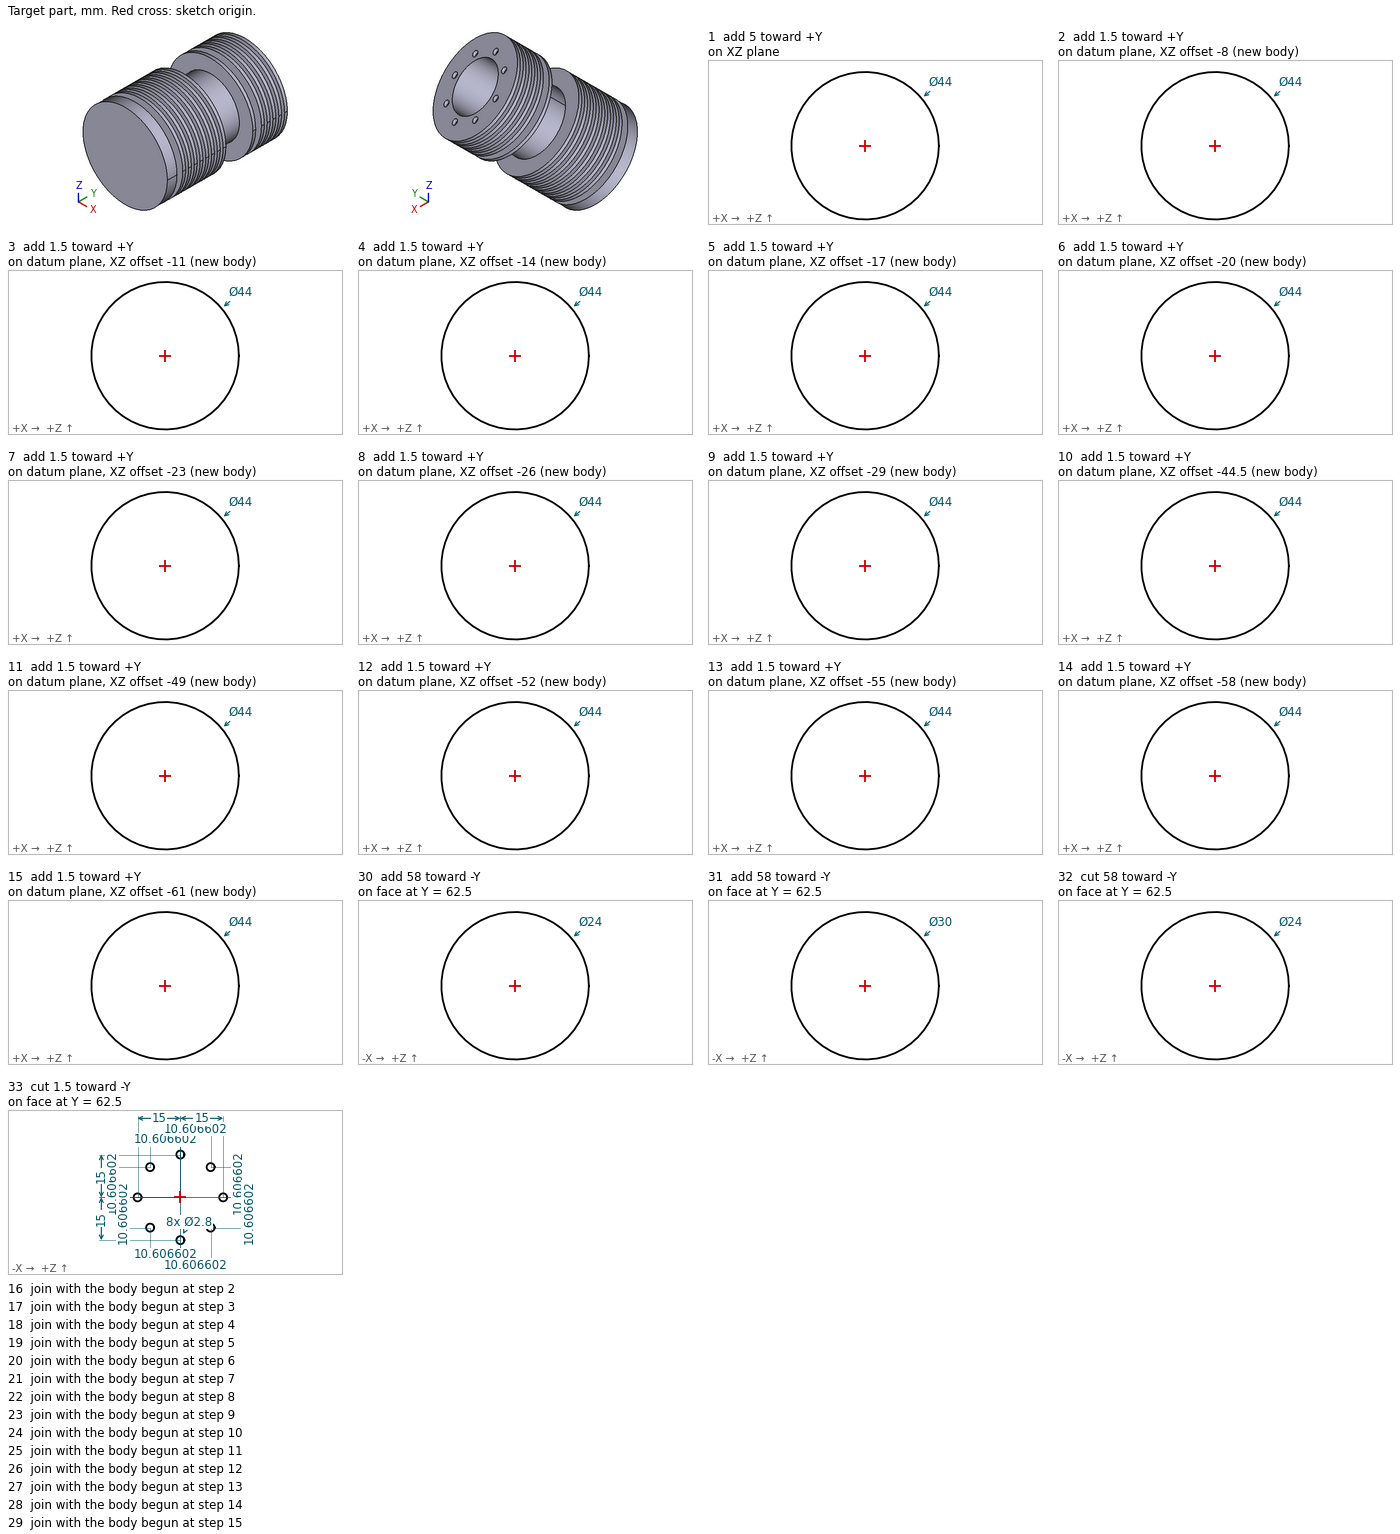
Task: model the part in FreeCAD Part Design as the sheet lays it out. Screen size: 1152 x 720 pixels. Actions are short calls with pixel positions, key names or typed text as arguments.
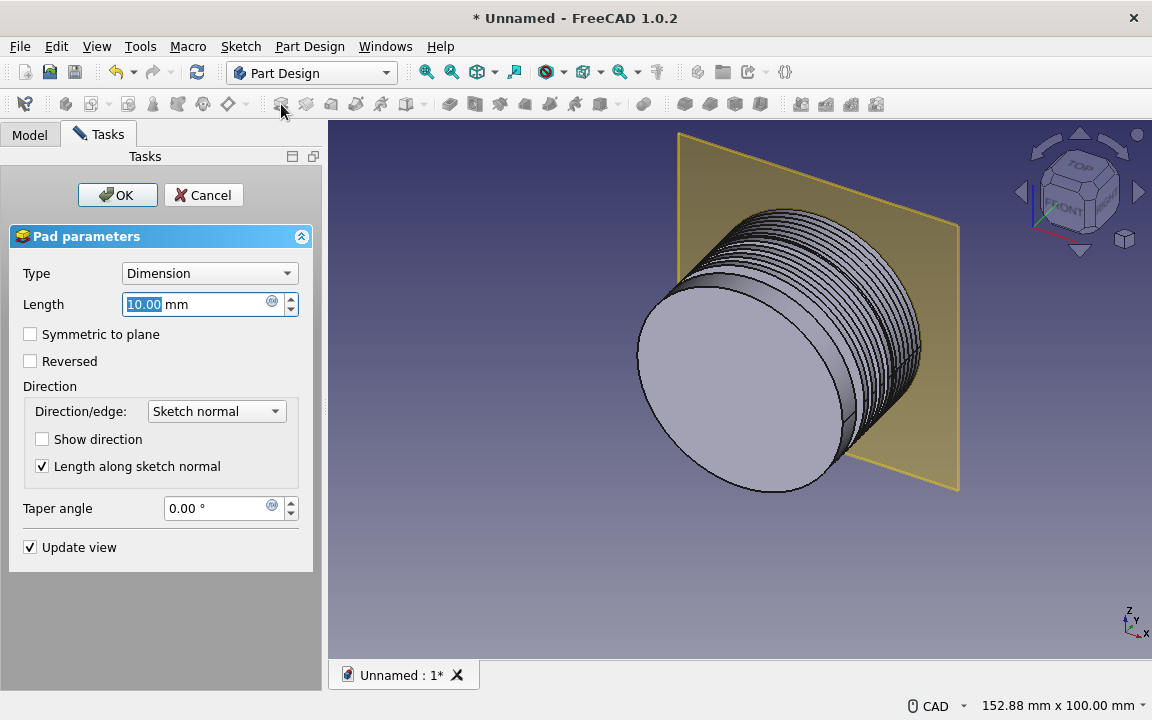
text(1.5)
key(Tab)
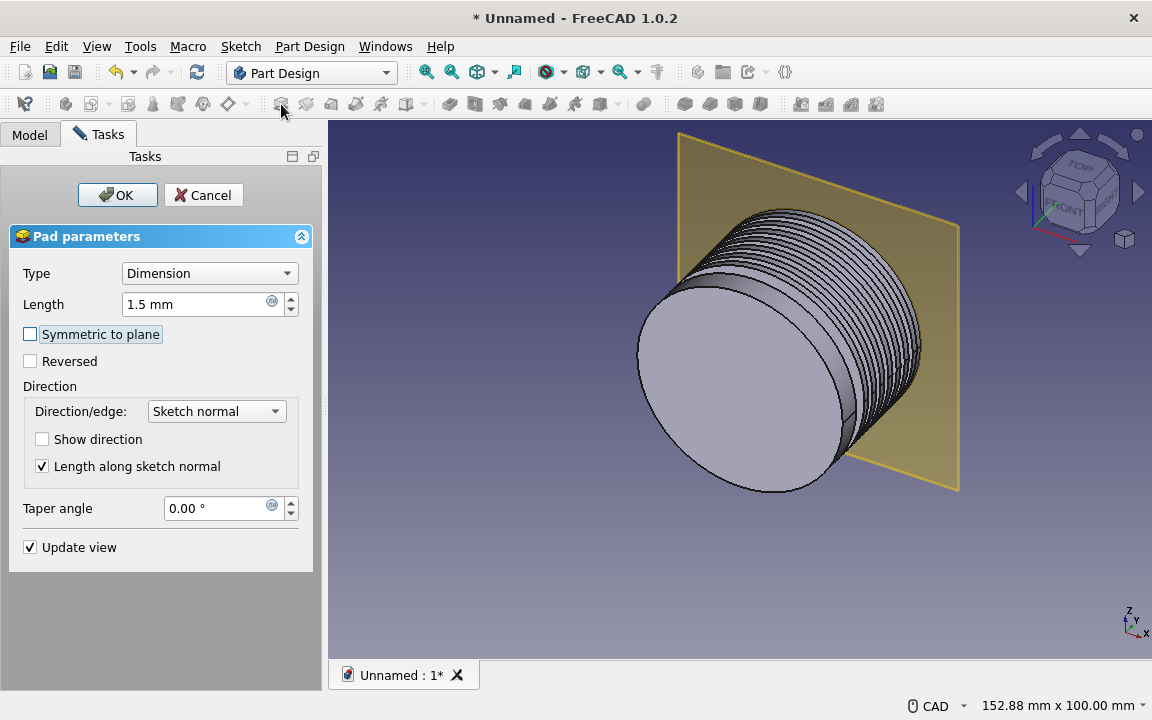
click(31, 361)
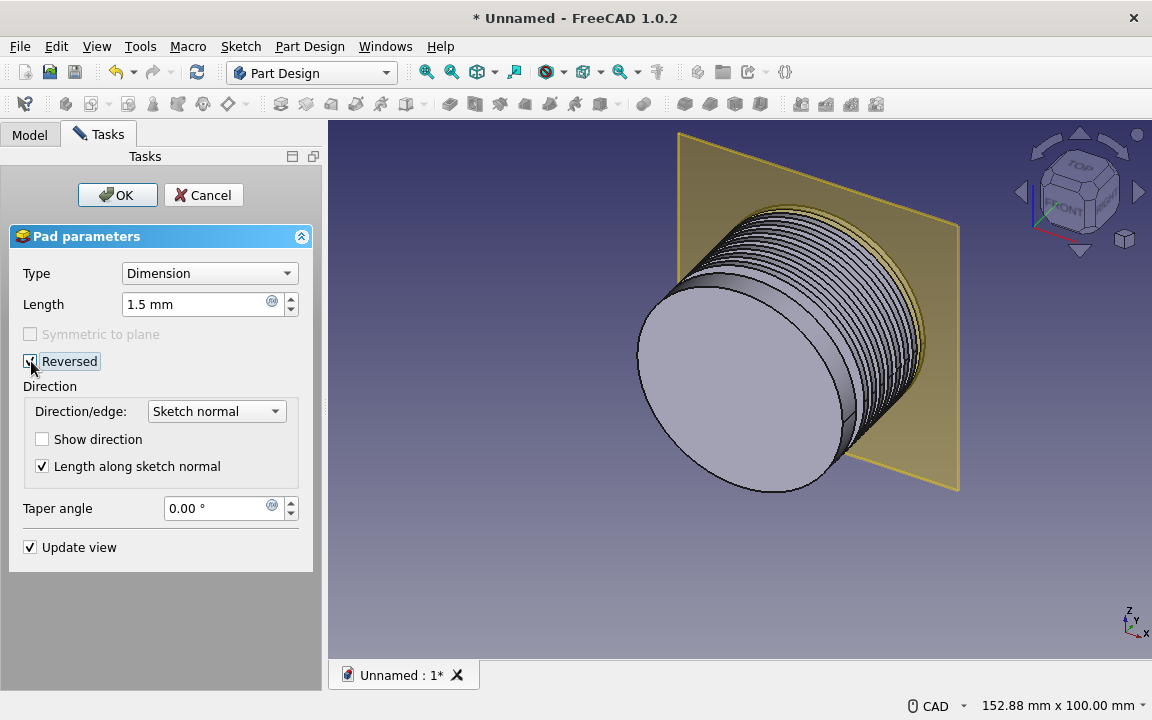
click(118, 195)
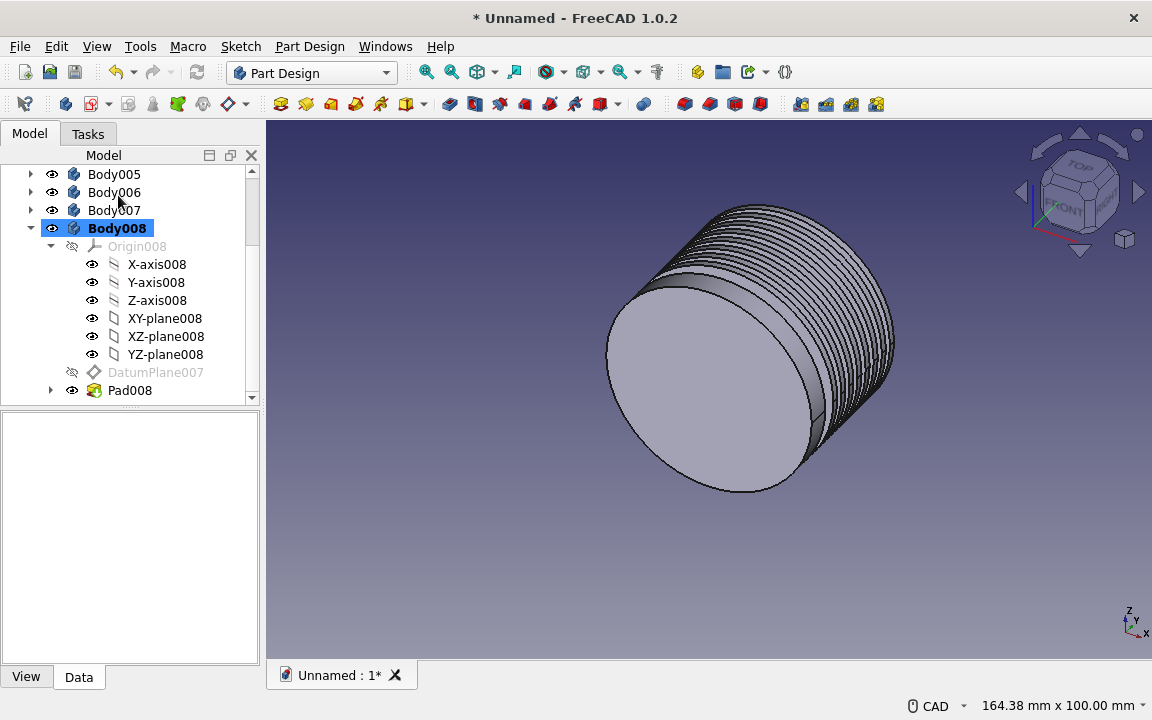
click(66, 104)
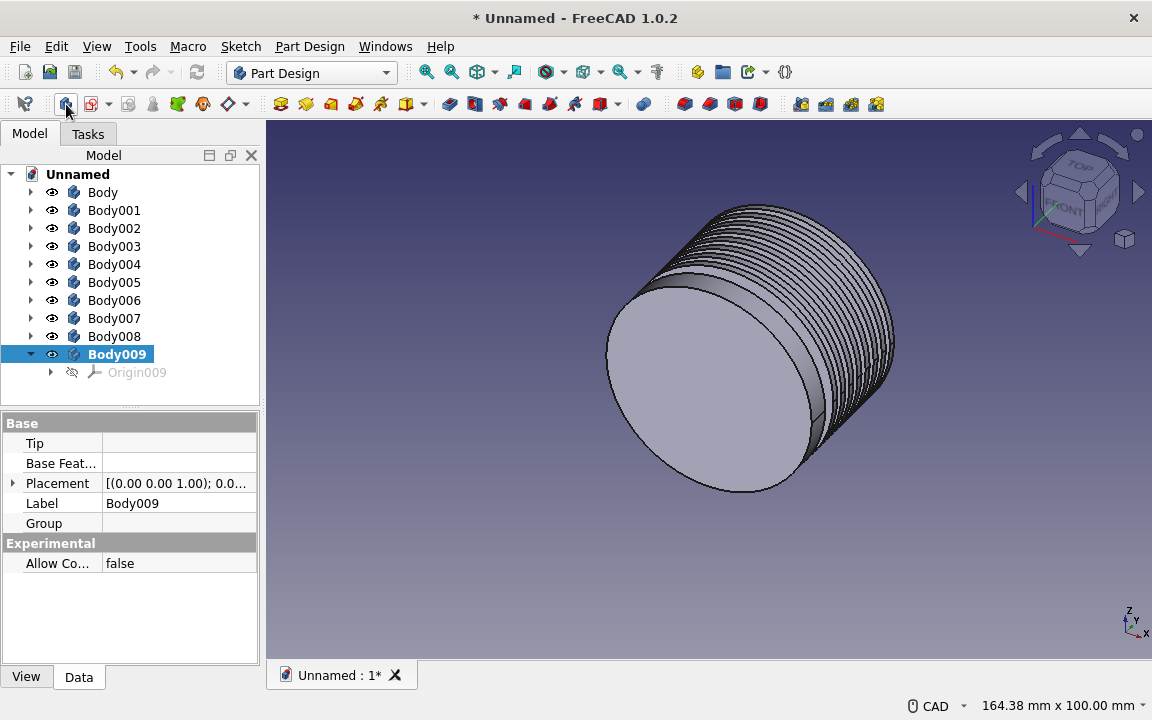
click(51, 372)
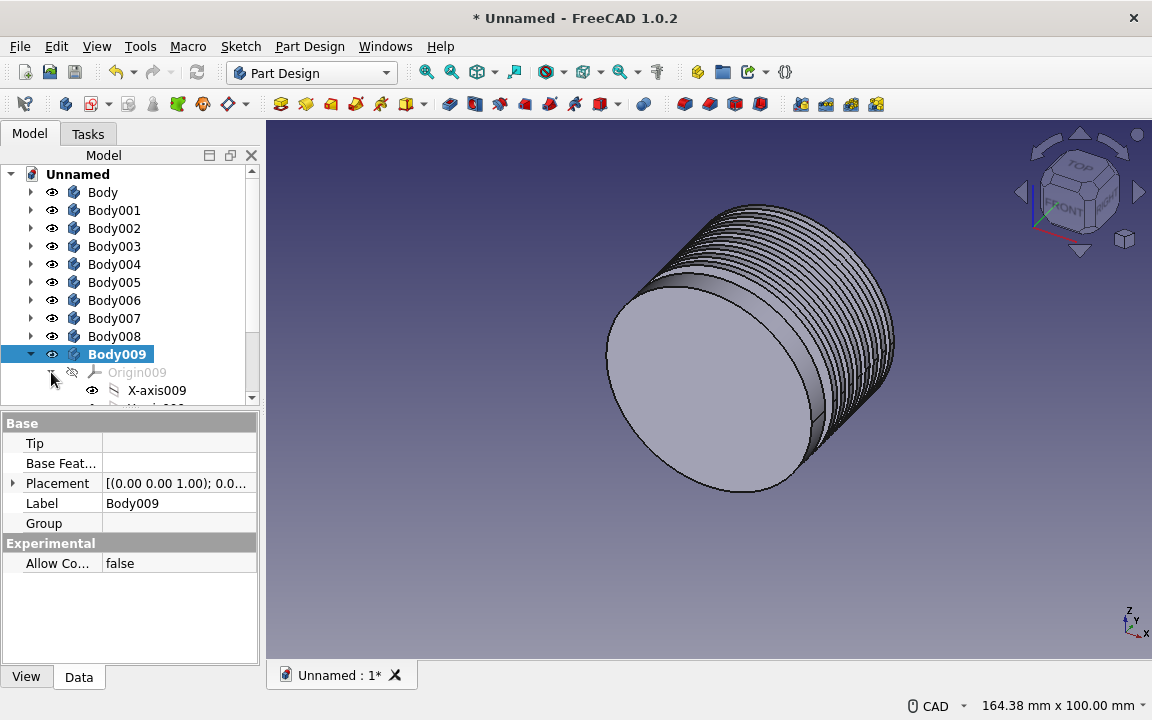
scroll(101, 278, down, 3)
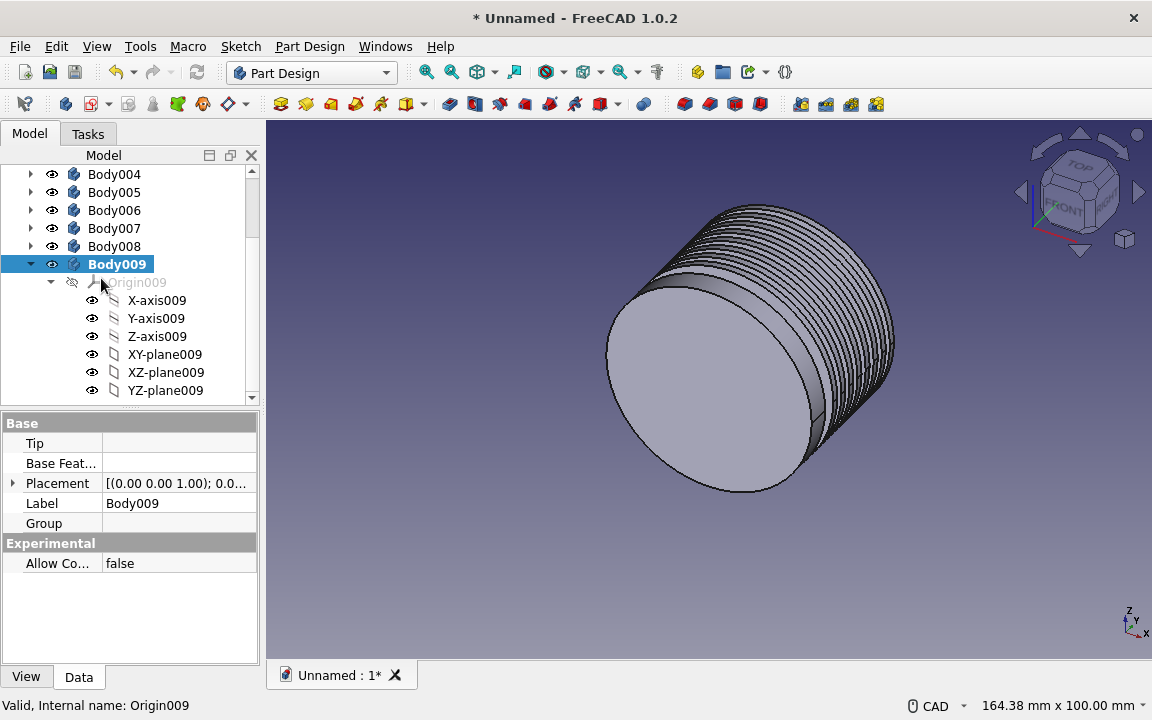
click(137, 372)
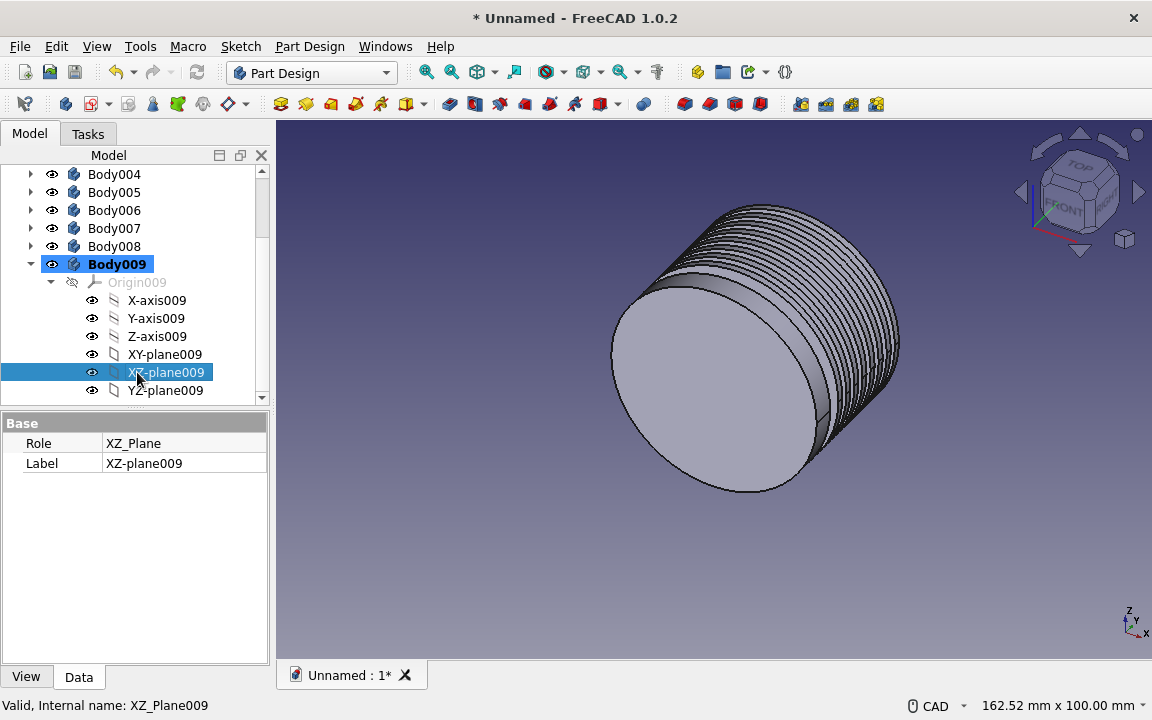
click(228, 104)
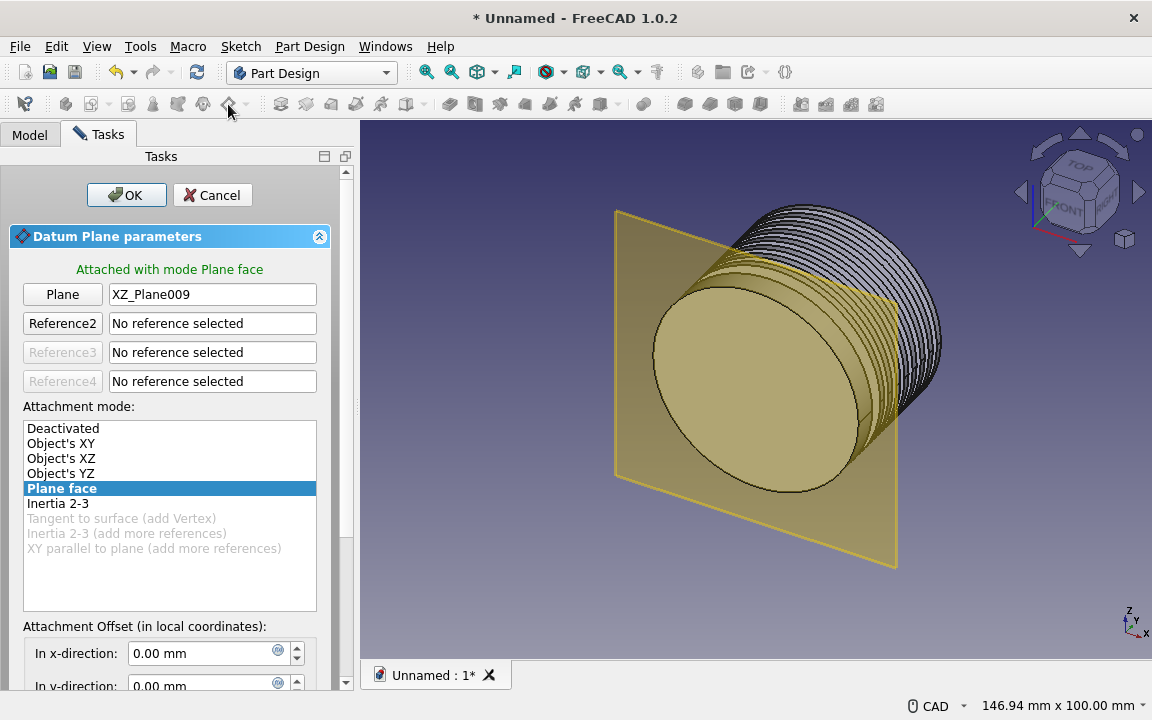
scroll(346, 428, down, 2)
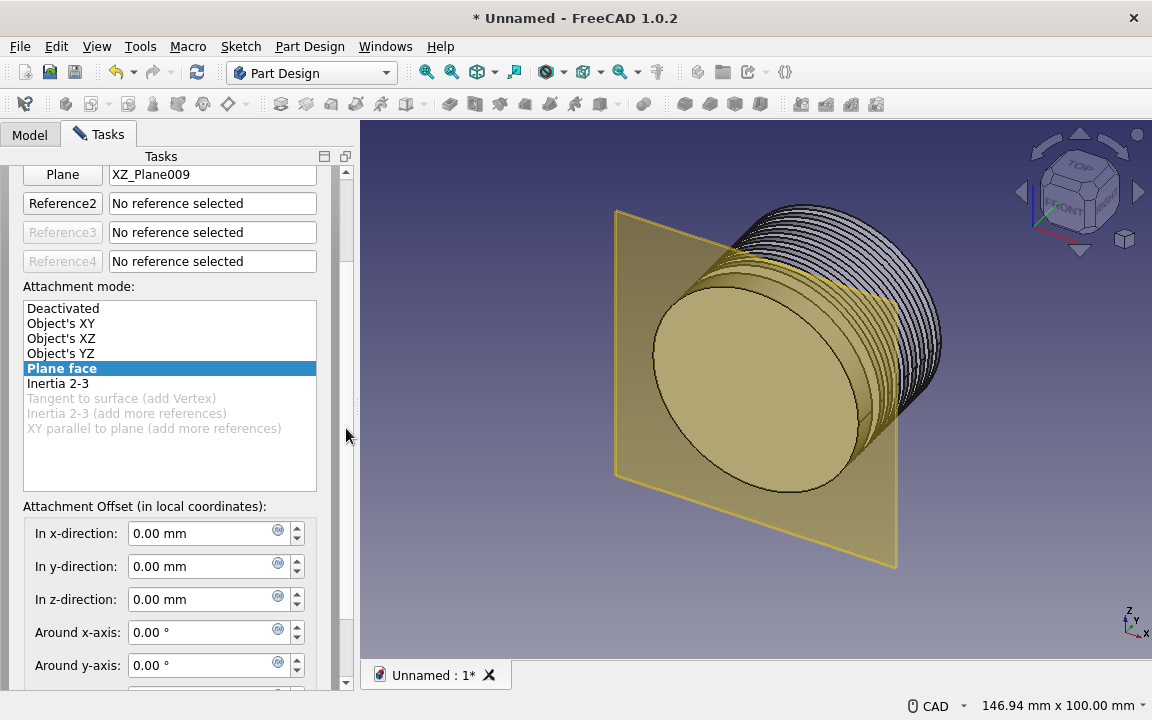
triple_click(210, 600)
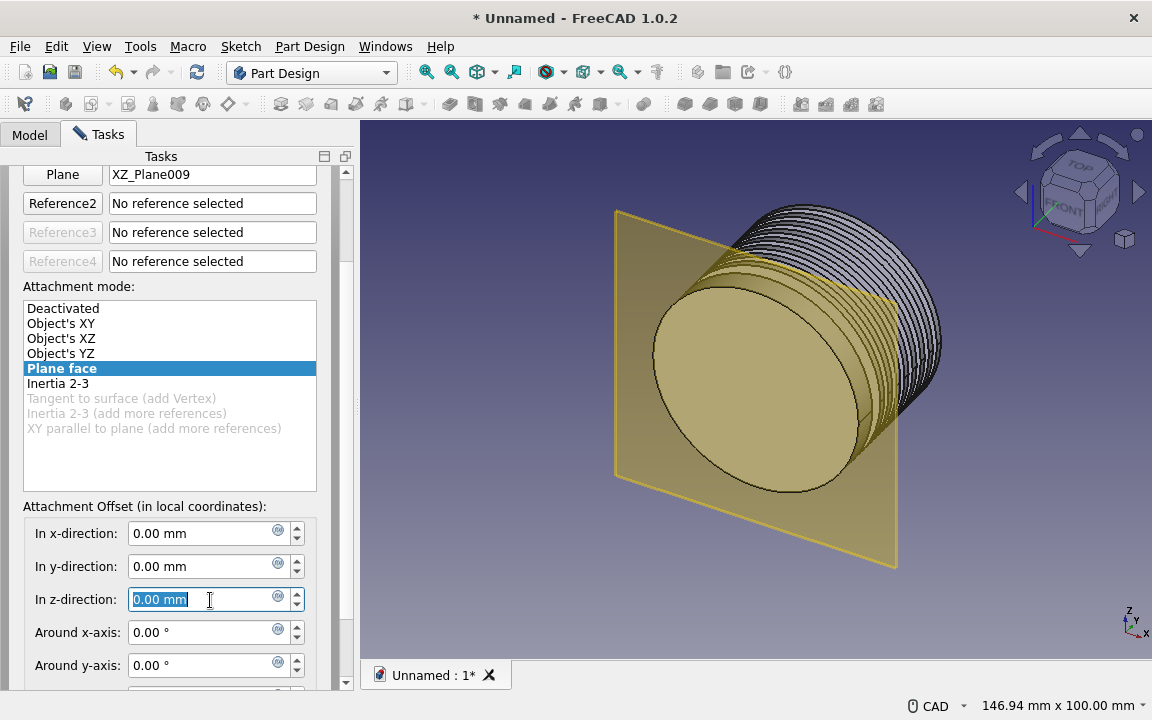
text(-44.5)
key(Tab)